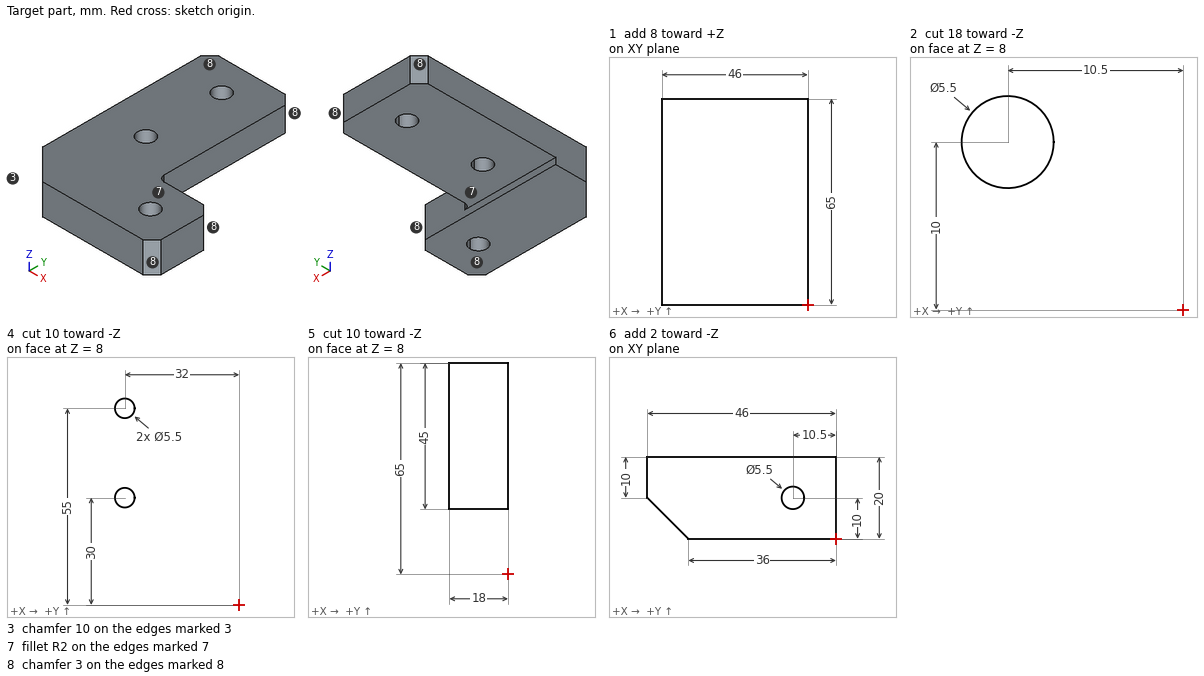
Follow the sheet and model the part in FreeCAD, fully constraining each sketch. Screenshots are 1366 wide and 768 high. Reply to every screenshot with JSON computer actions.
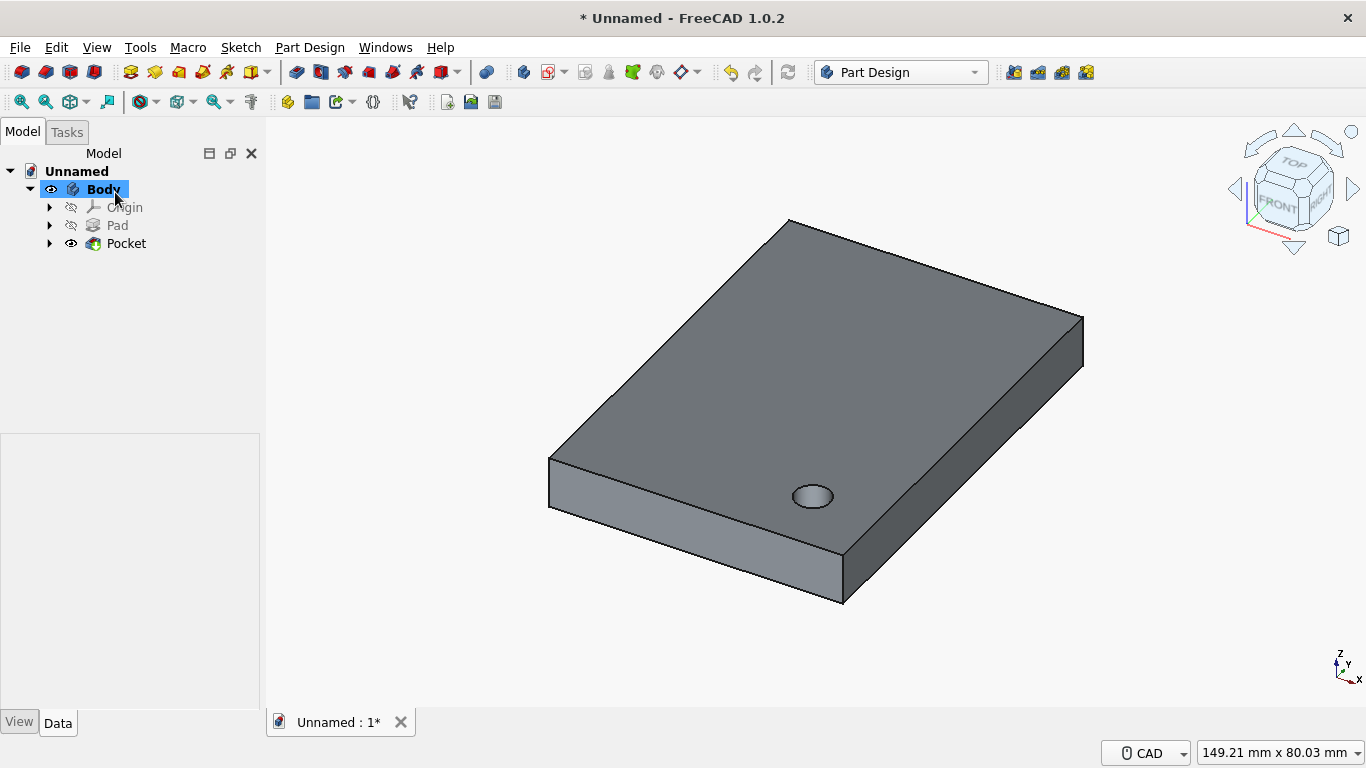
{"action": "key", "text": "0"}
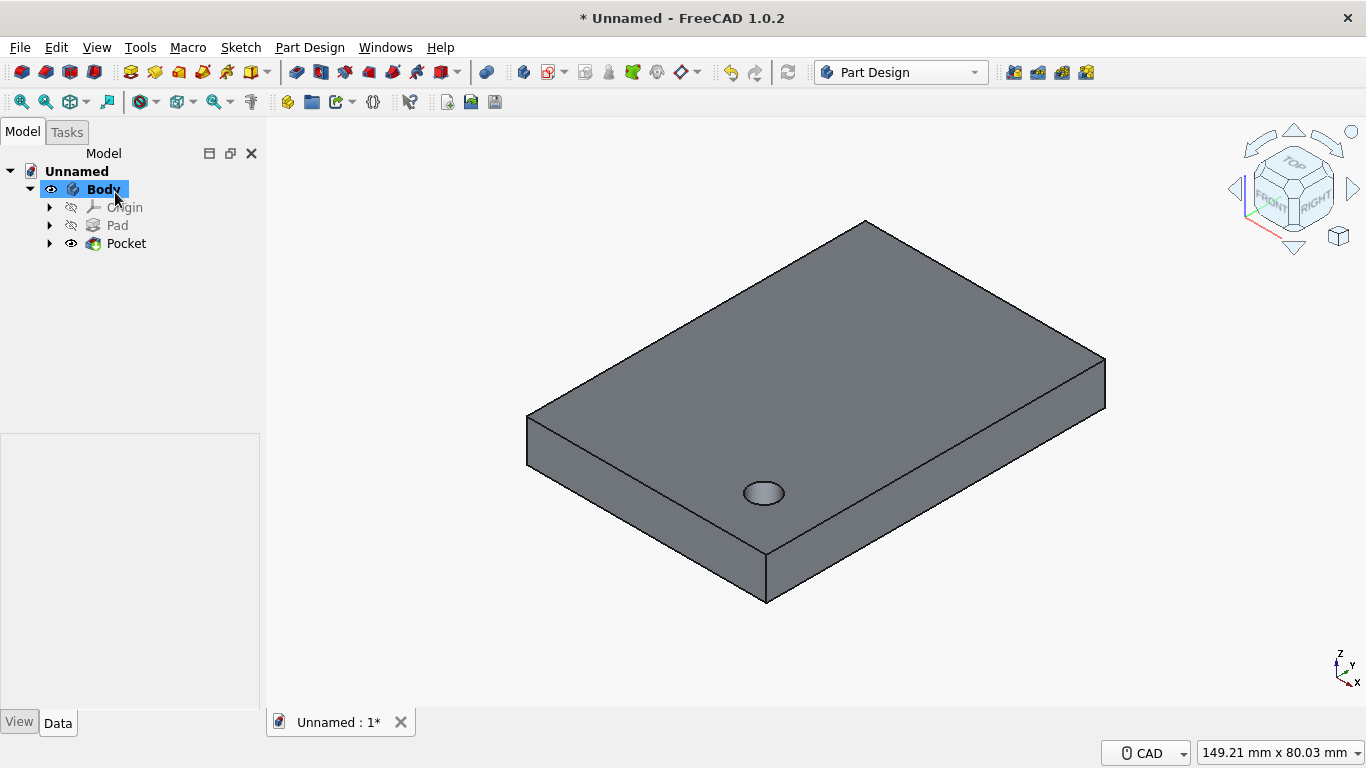
{"action": "key", "text": "2"}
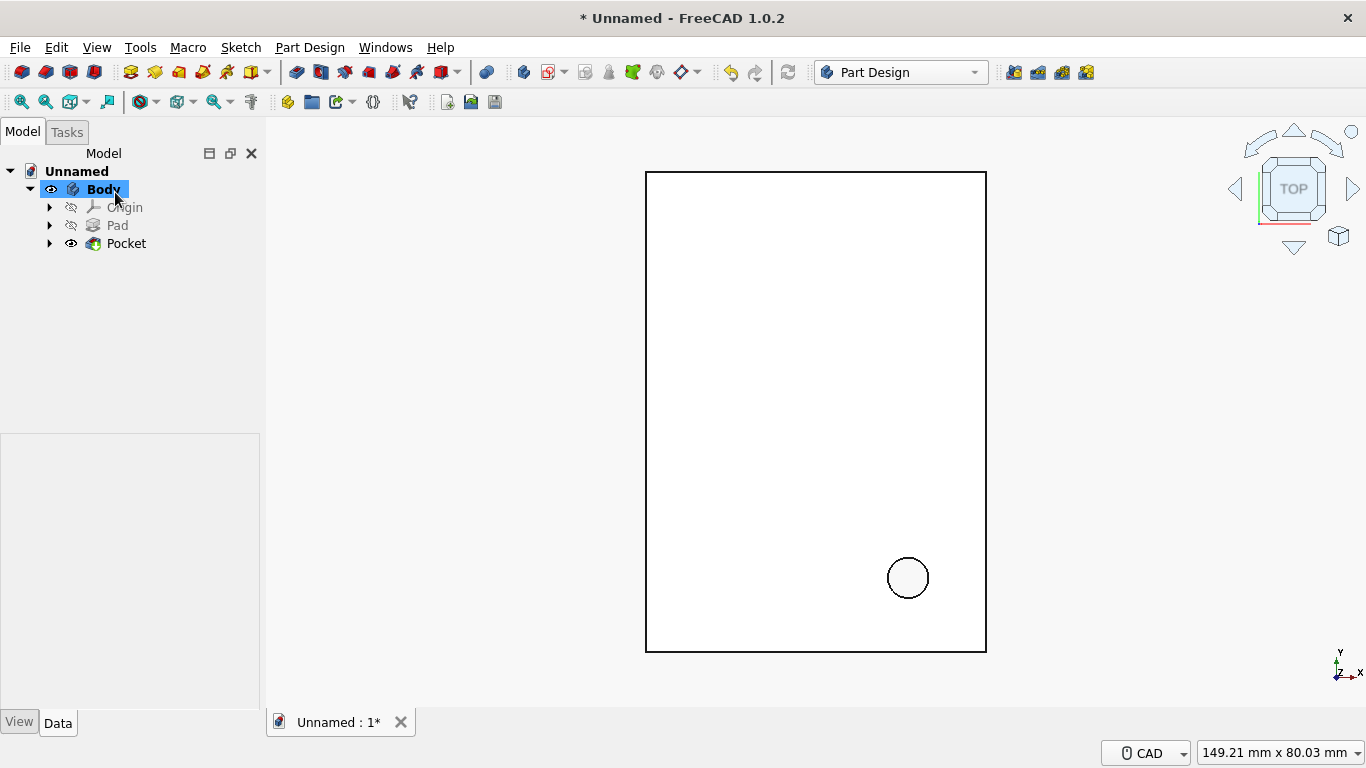
{"action": "key", "text": "1"}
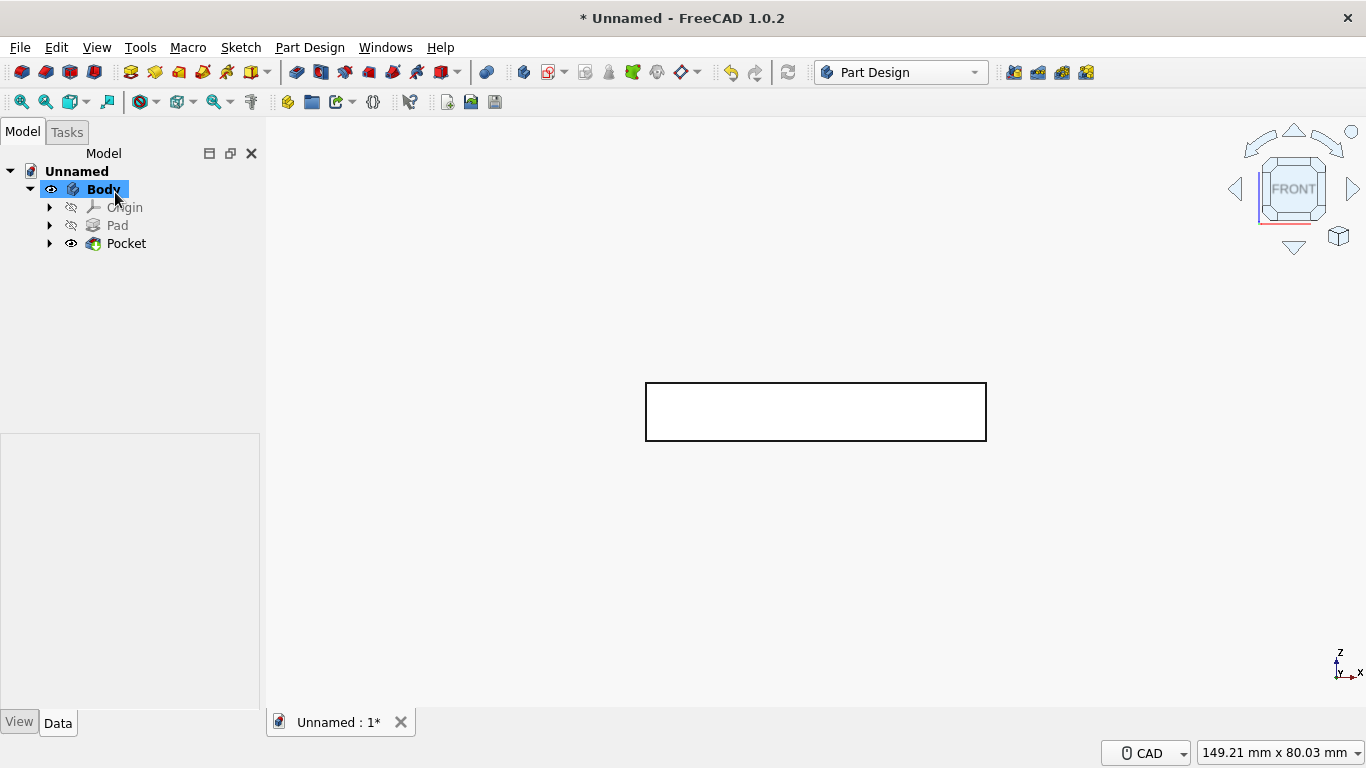
{"action": "left_click", "coordinate": [22, 102]}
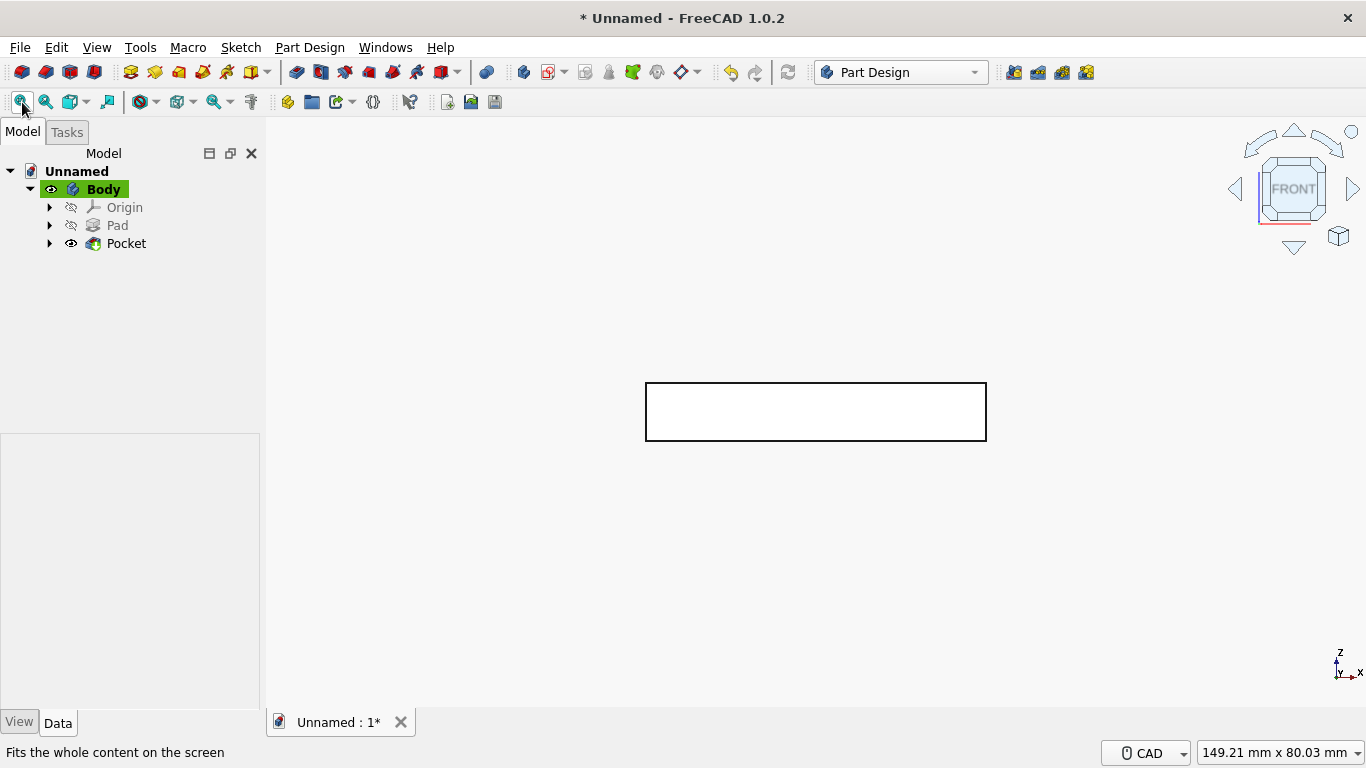
{"action": "left_click", "coordinate": [646, 411]}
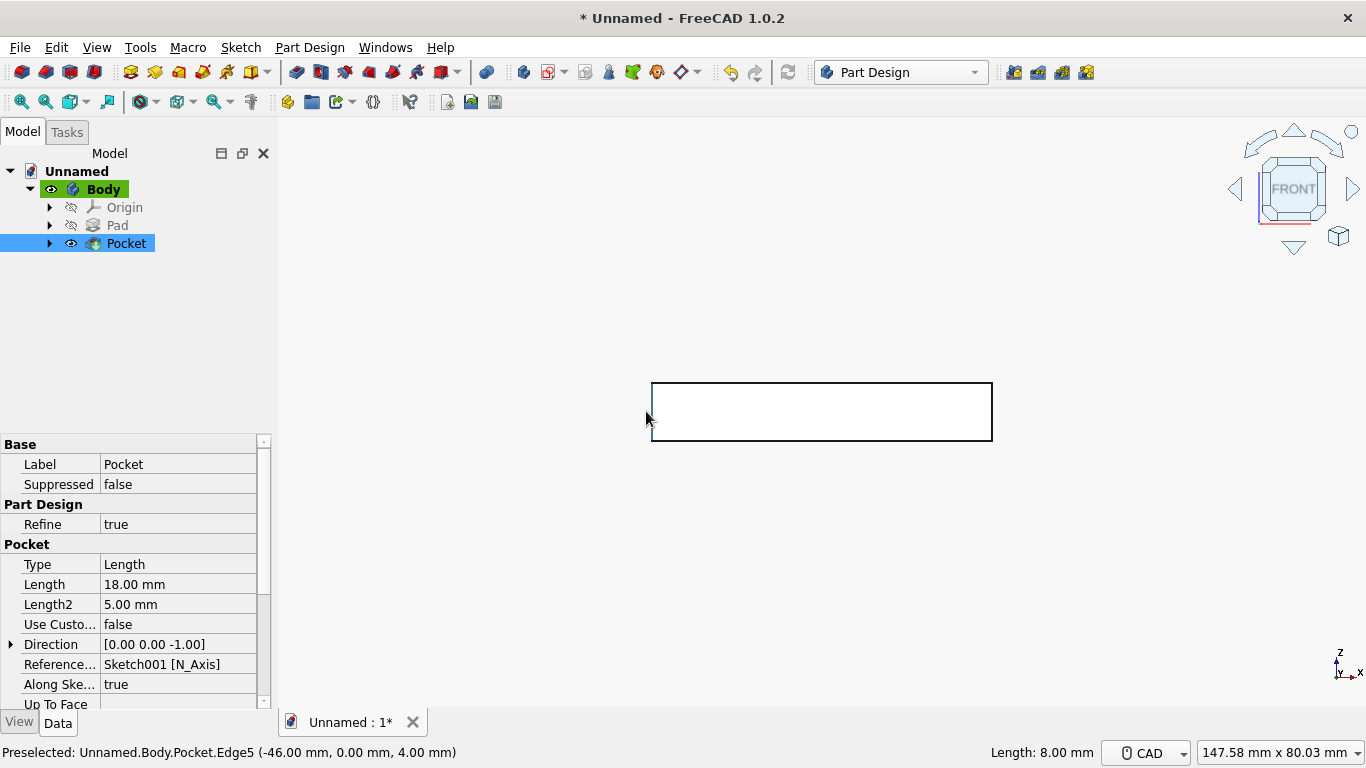
{"action": "left_click", "coordinate": [46, 72]}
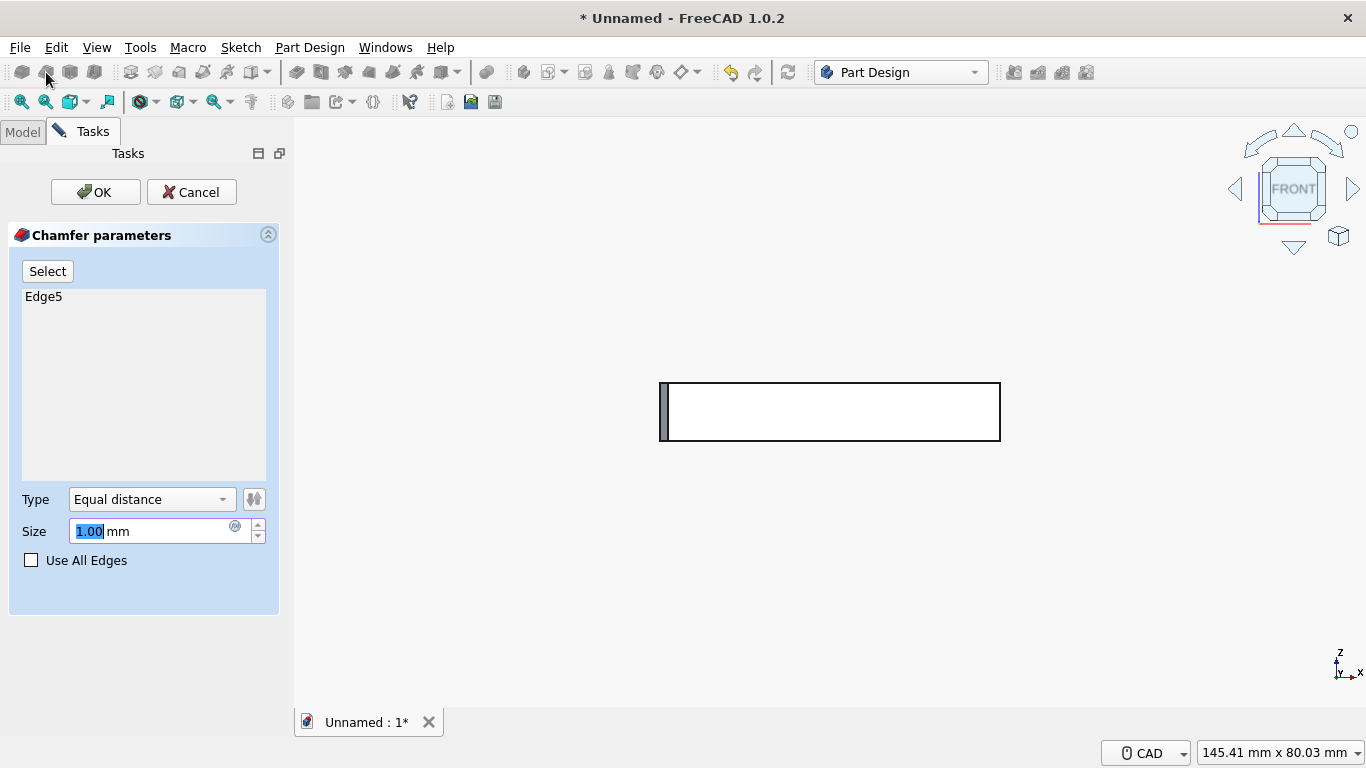
{"action": "type", "text": "10"}
{"action": "key", "text": "Tab"}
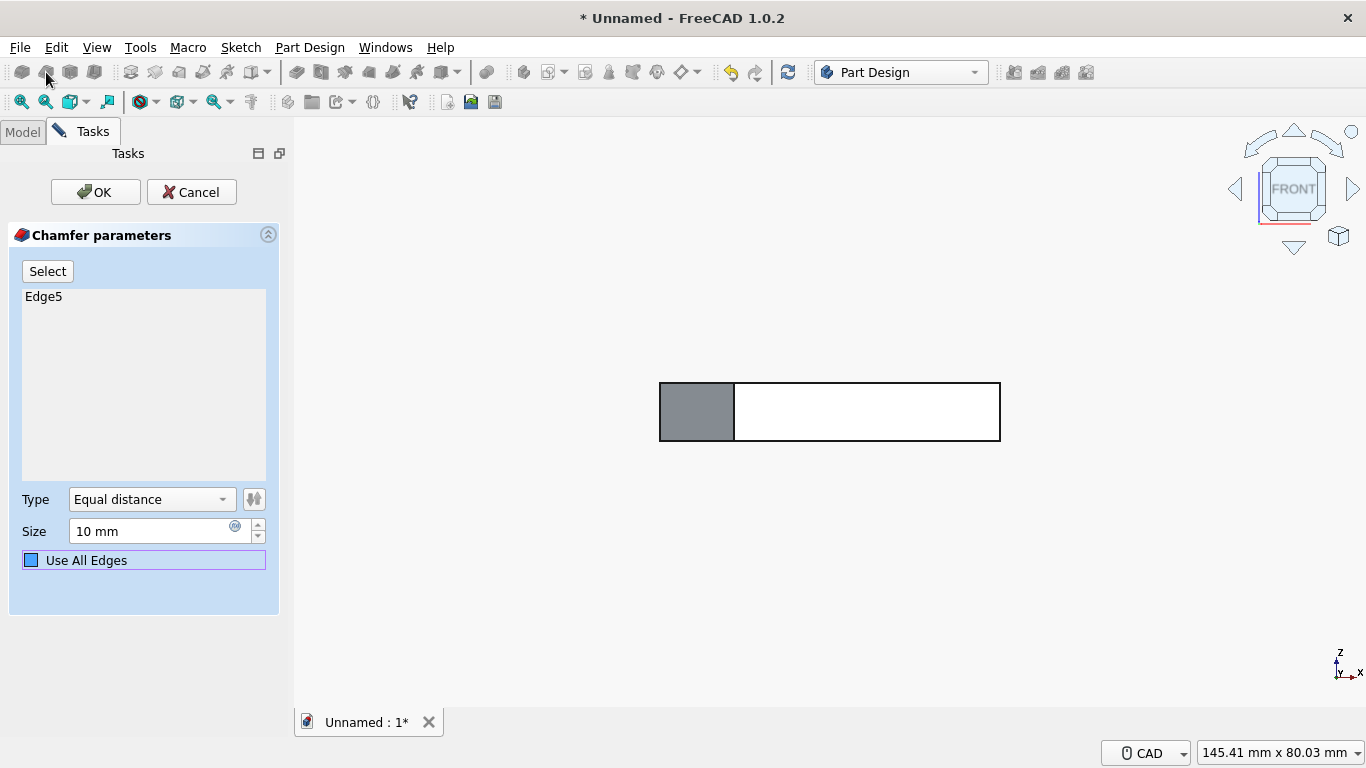
{"action": "left_click", "coordinate": [96, 192]}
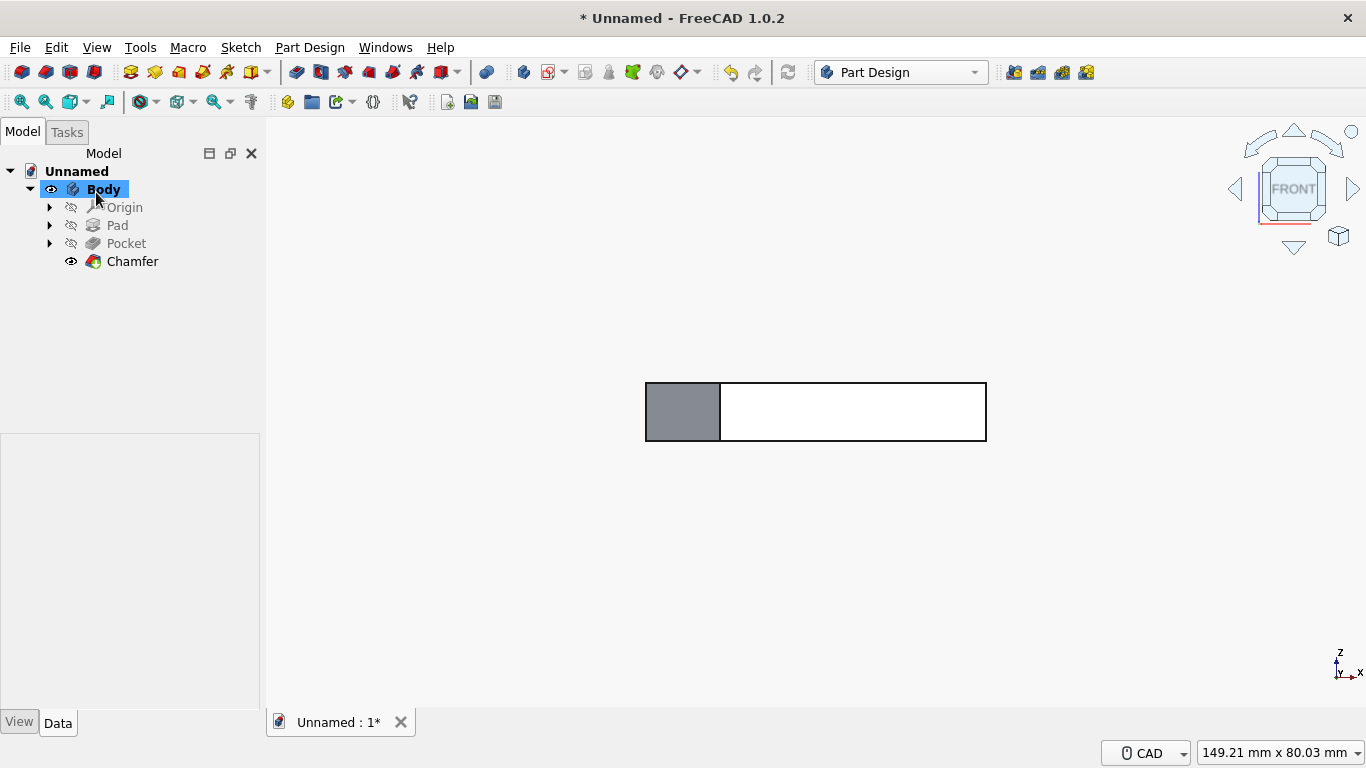
{"action": "key", "text": "v f"}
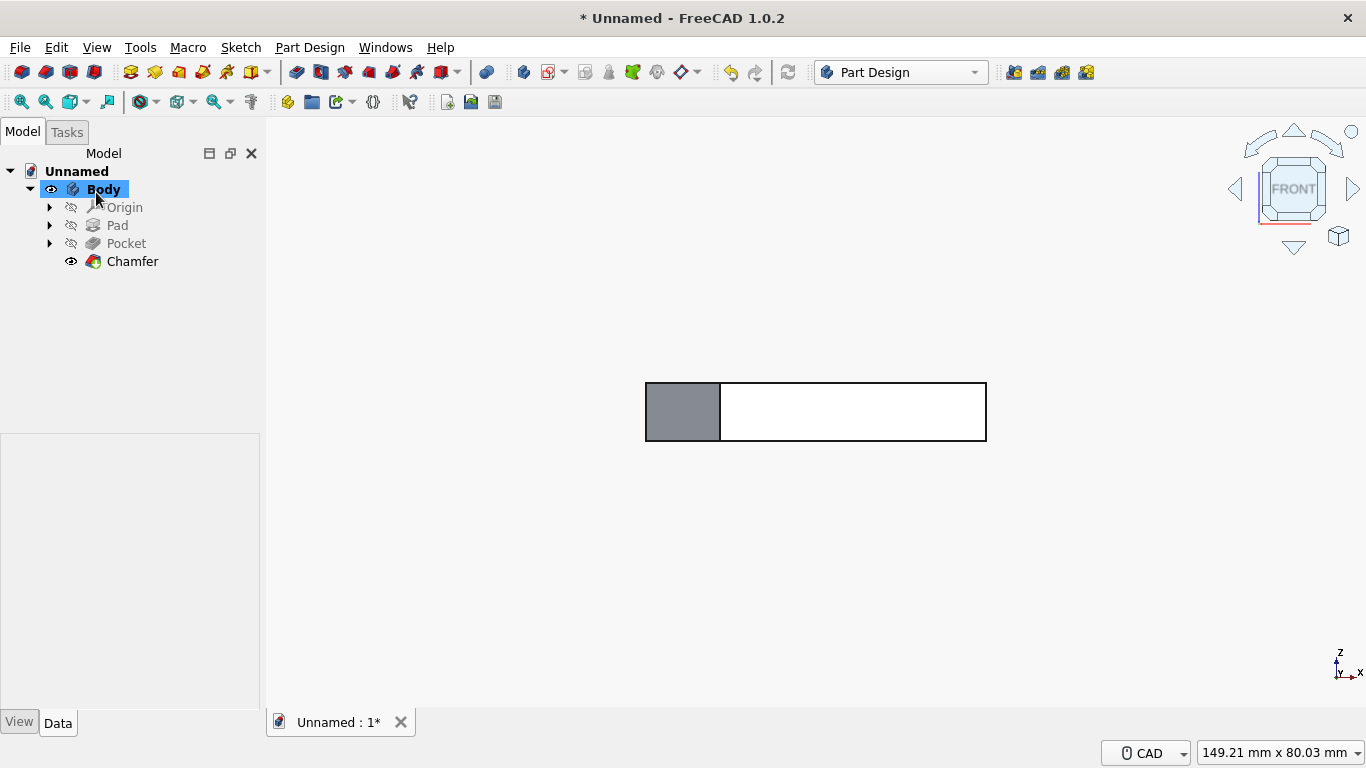
{"action": "key", "text": "0"}